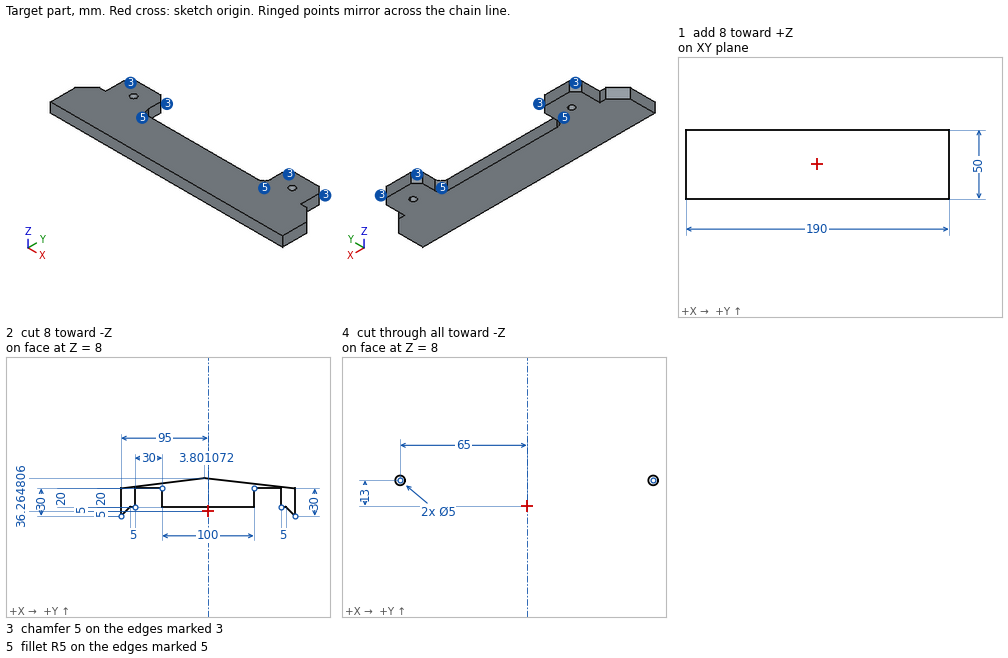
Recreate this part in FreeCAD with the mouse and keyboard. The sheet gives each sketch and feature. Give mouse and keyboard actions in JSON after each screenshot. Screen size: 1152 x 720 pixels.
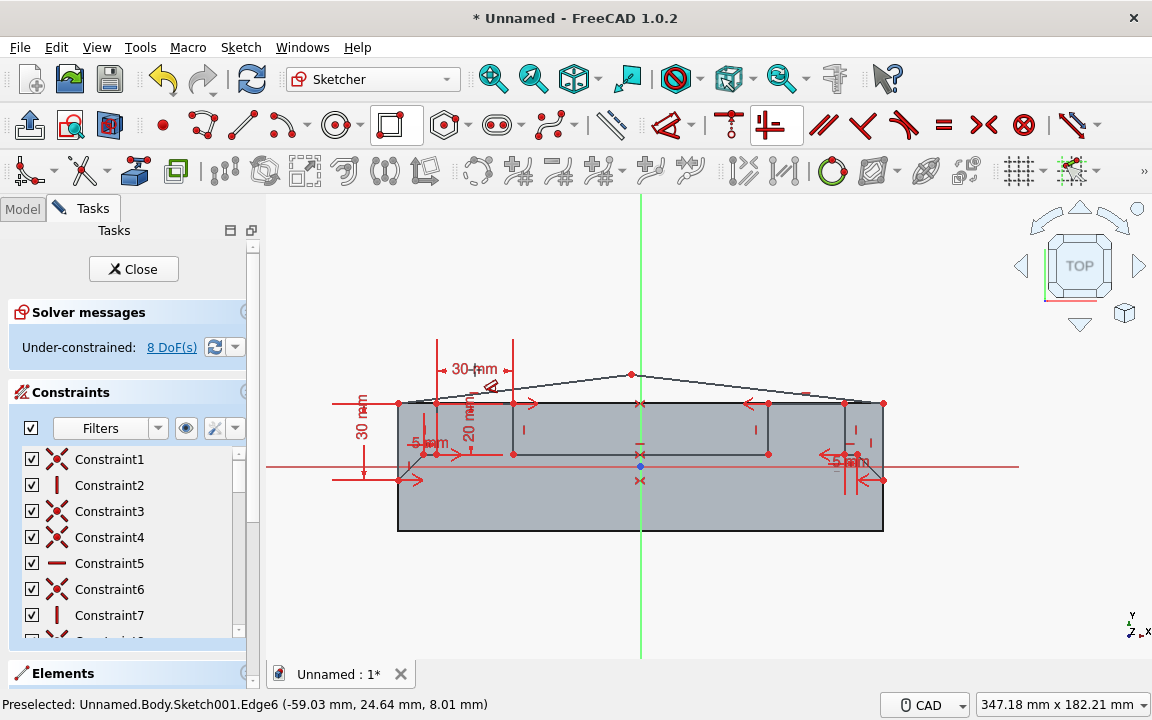
{"action": "left_click", "coordinate": [513, 419]}
{"action": "left_click", "coordinate": [547, 429]}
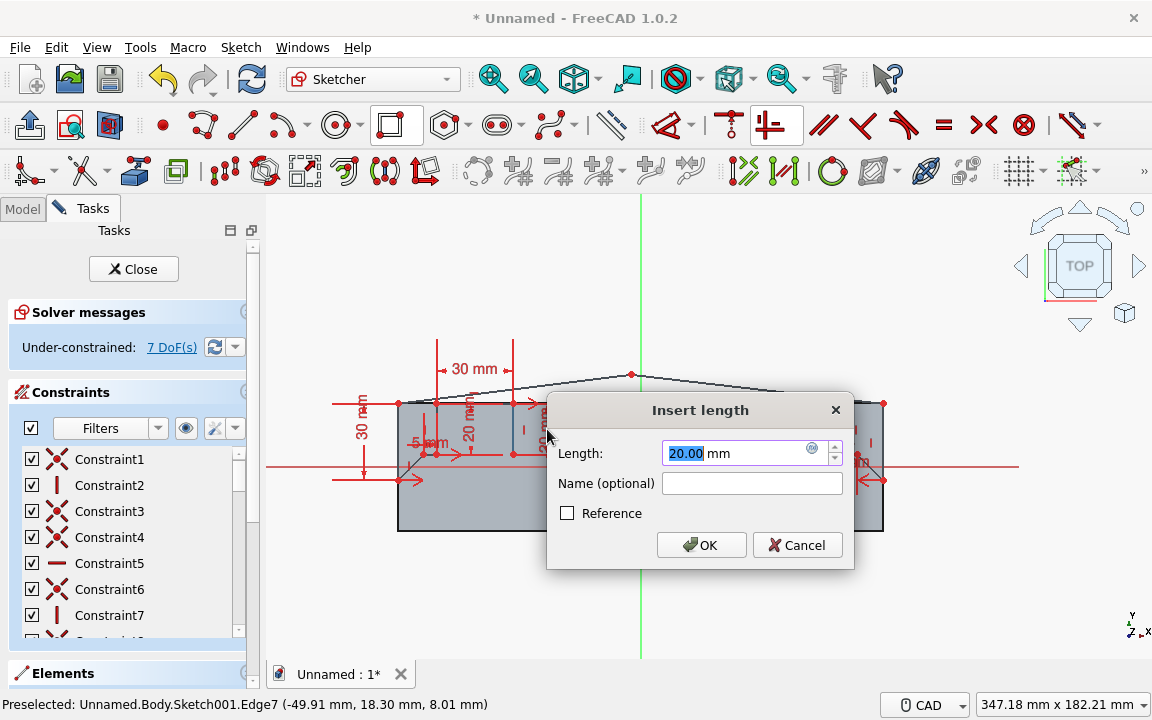
{"action": "type", "text": "20"}
{"action": "key", "text": "Return"}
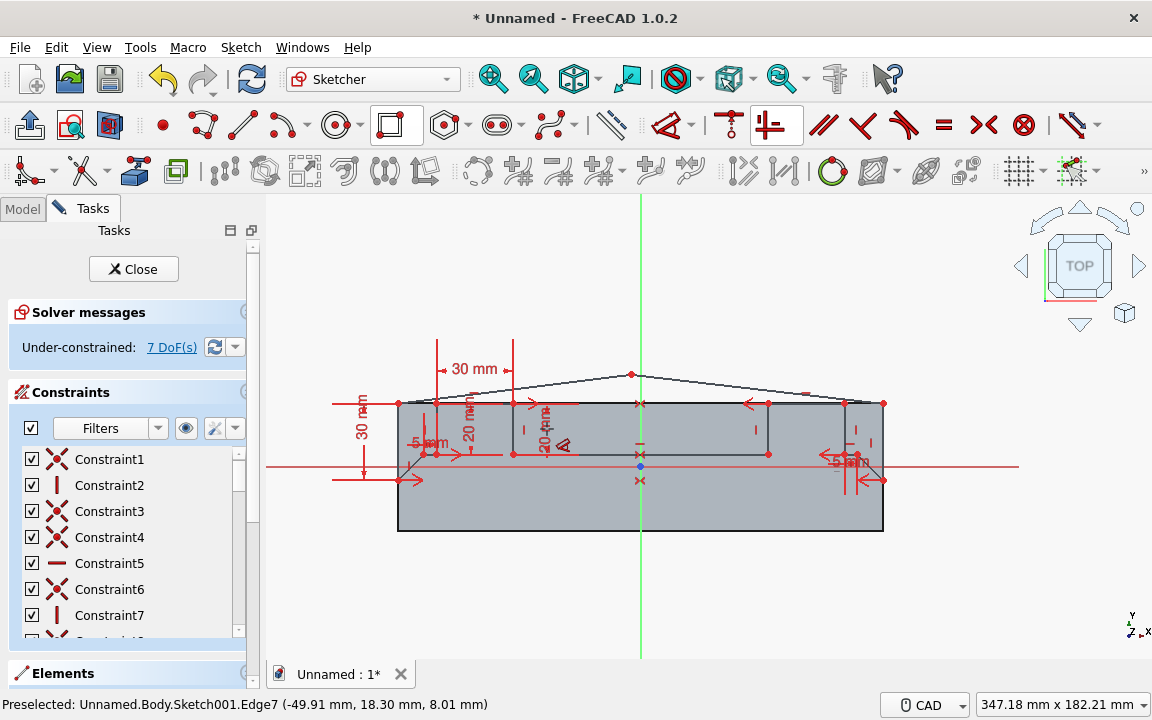
{"action": "scroll", "coordinate": [883, 457], "scroll_direction": "up", "scroll_amount": 2}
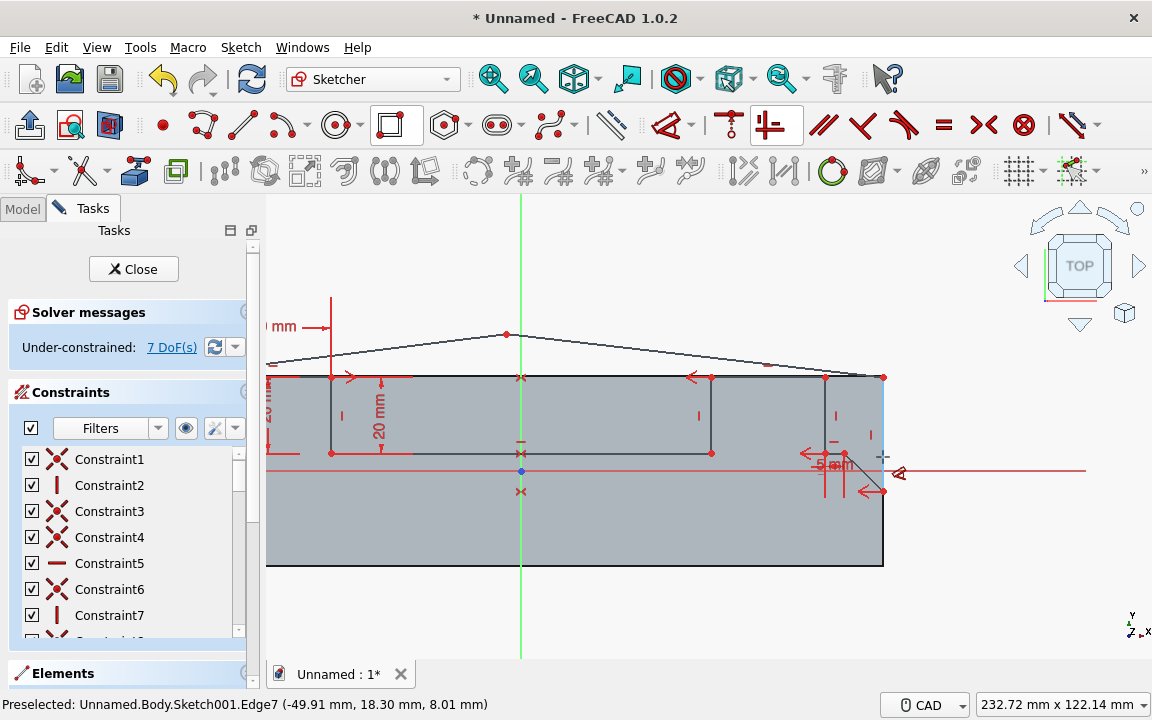
{"action": "left_click", "coordinate": [883, 457]}
{"action": "left_click", "coordinate": [917, 435]}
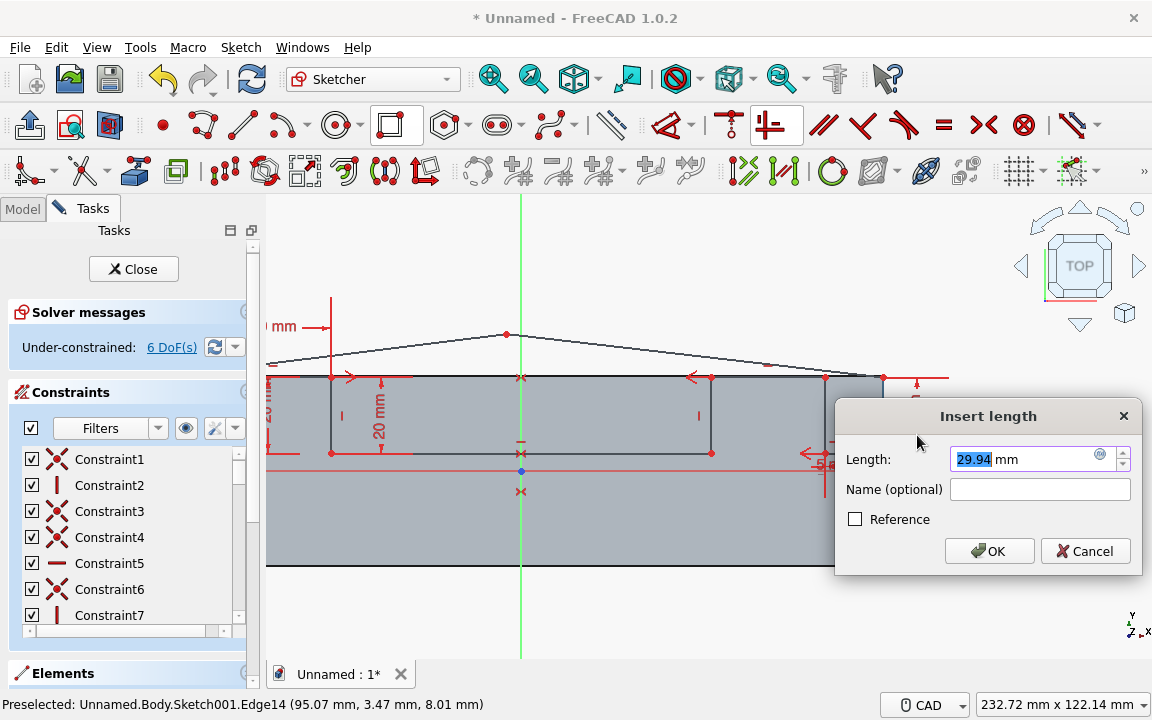
{"action": "type", "text": "30"}
{"action": "key", "text": "Return"}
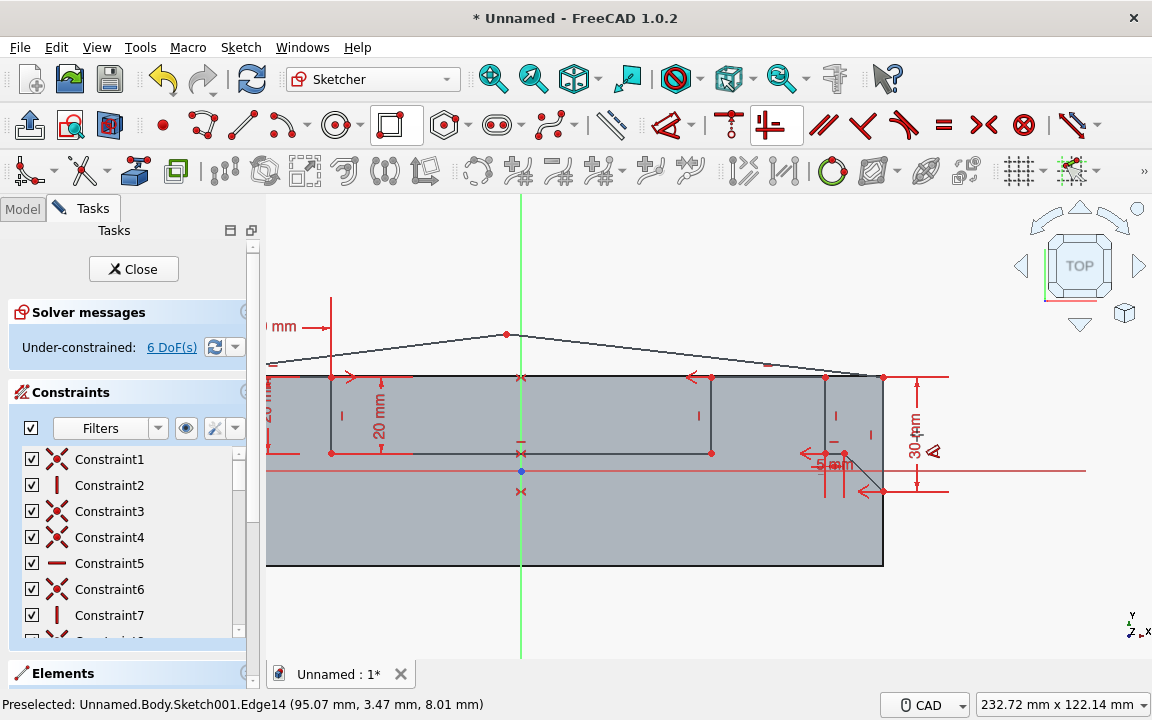
{"action": "scroll", "coordinate": [883, 457], "scroll_direction": "down", "scroll_amount": 2}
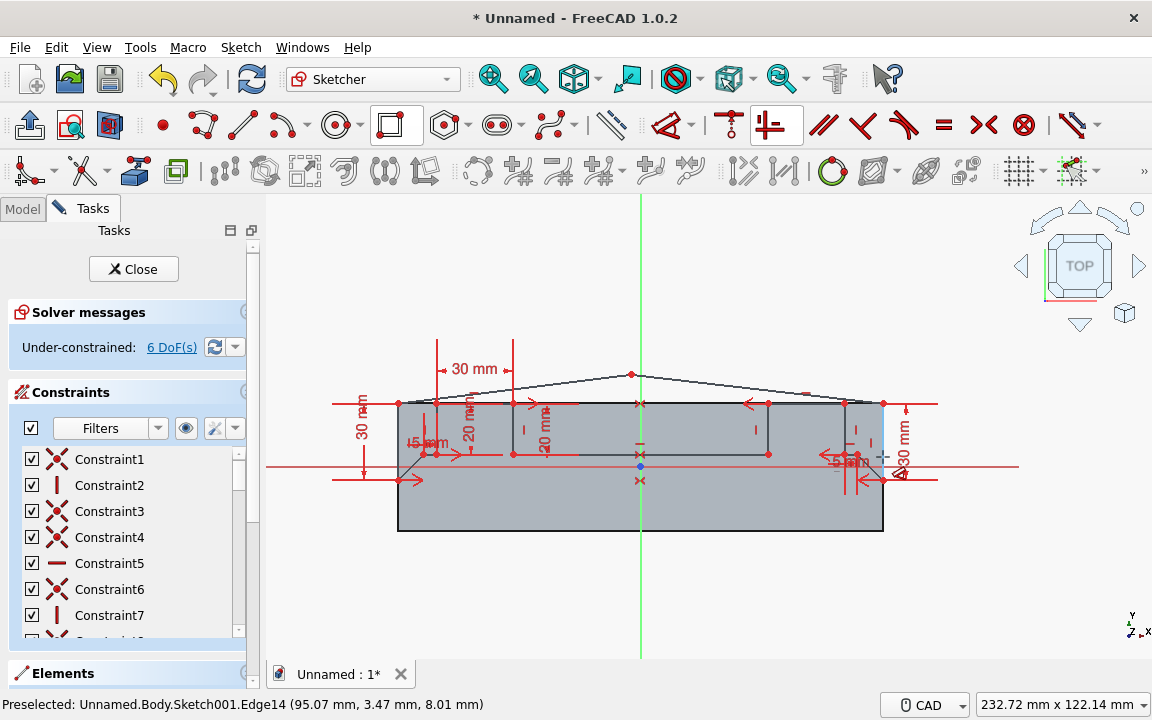
{"action": "scroll", "coordinate": [398, 480], "scroll_direction": "up", "scroll_amount": 6}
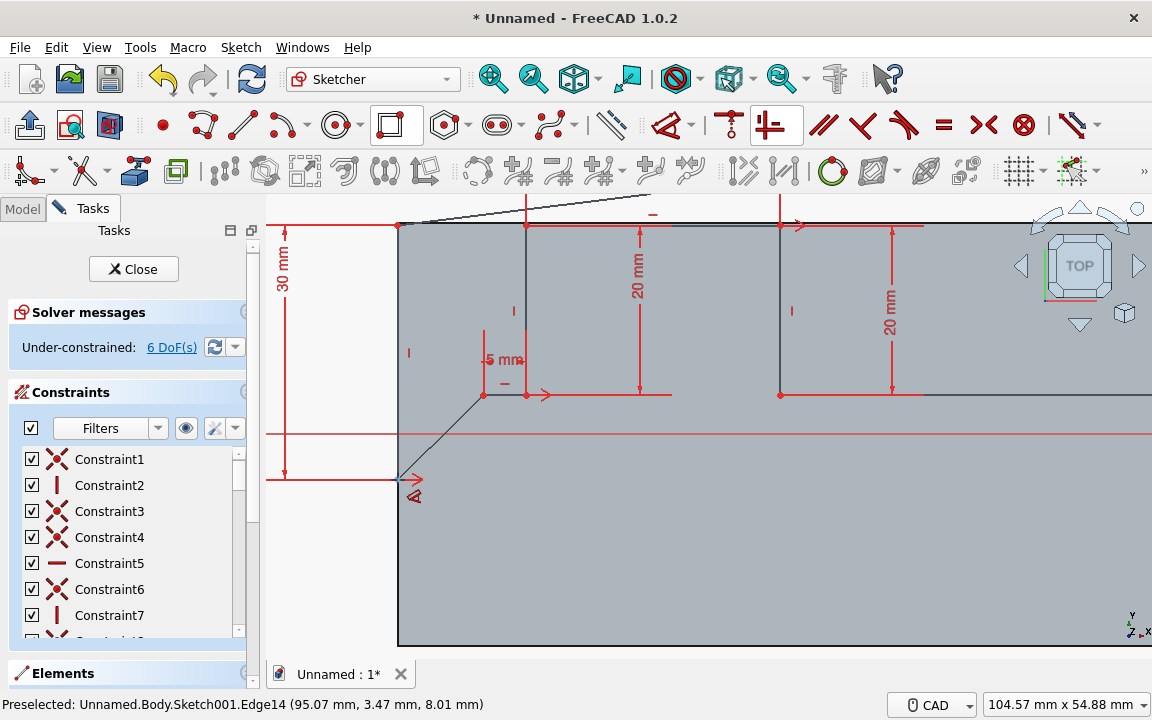
{"action": "left_click", "coordinate": [398, 480]}
{"action": "left_click", "coordinate": [364, 457]}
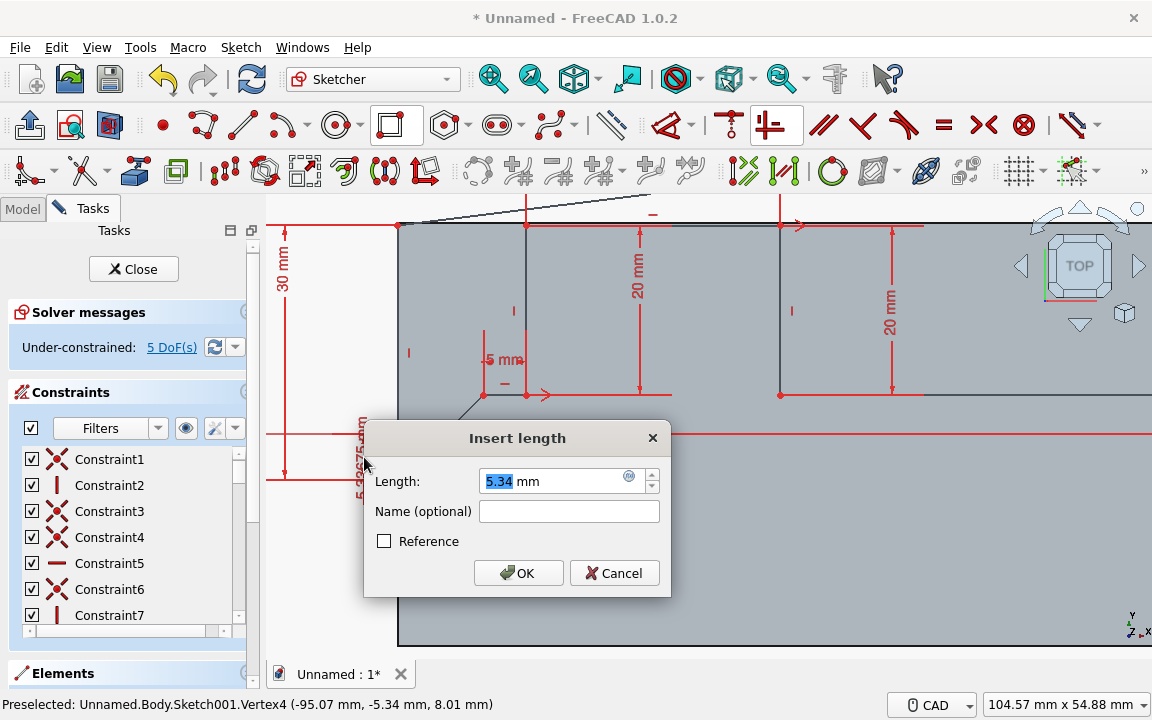
{"action": "type", "text": "5"}
{"action": "key", "text": "Return"}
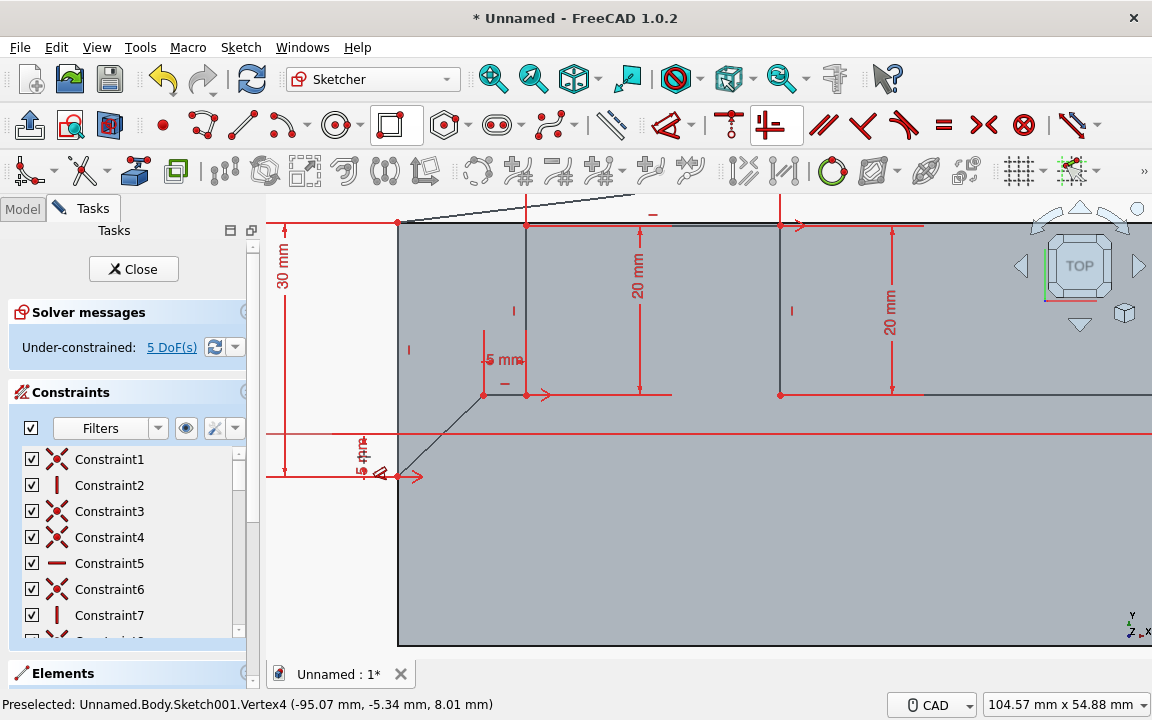
{"action": "left_click", "coordinate": [484, 395]}
{"action": "left_click", "coordinate": [450, 406]}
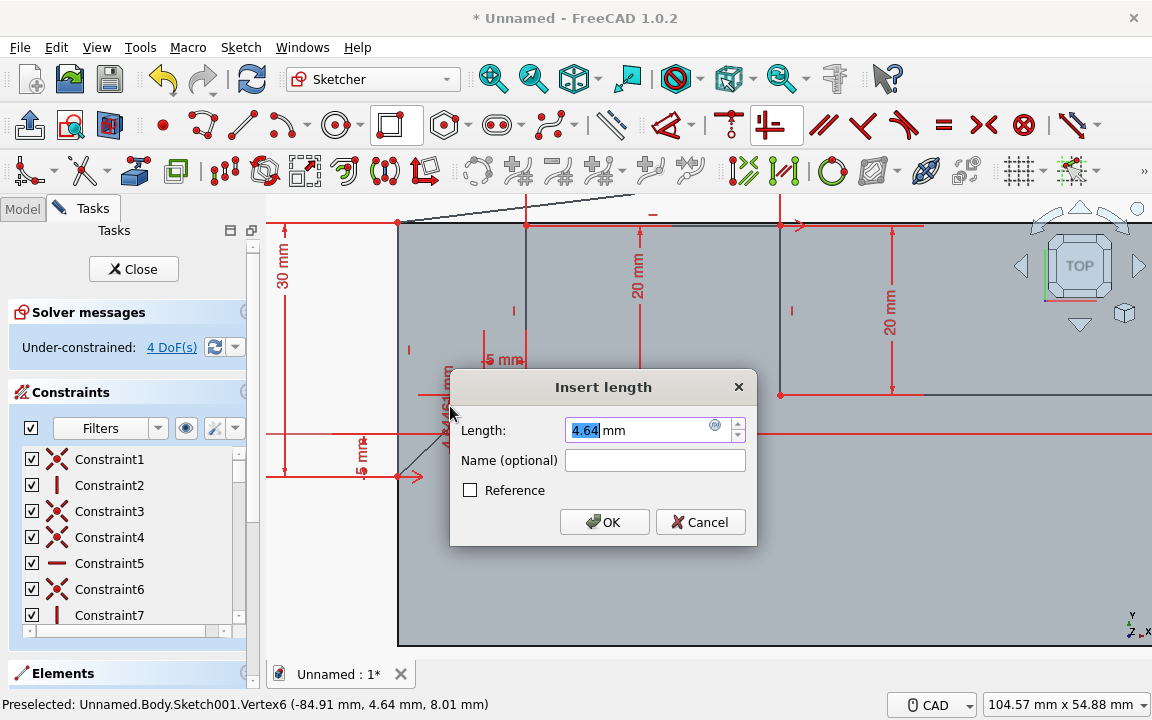
{"action": "type", "text": "5"}
{"action": "key", "text": "Return"}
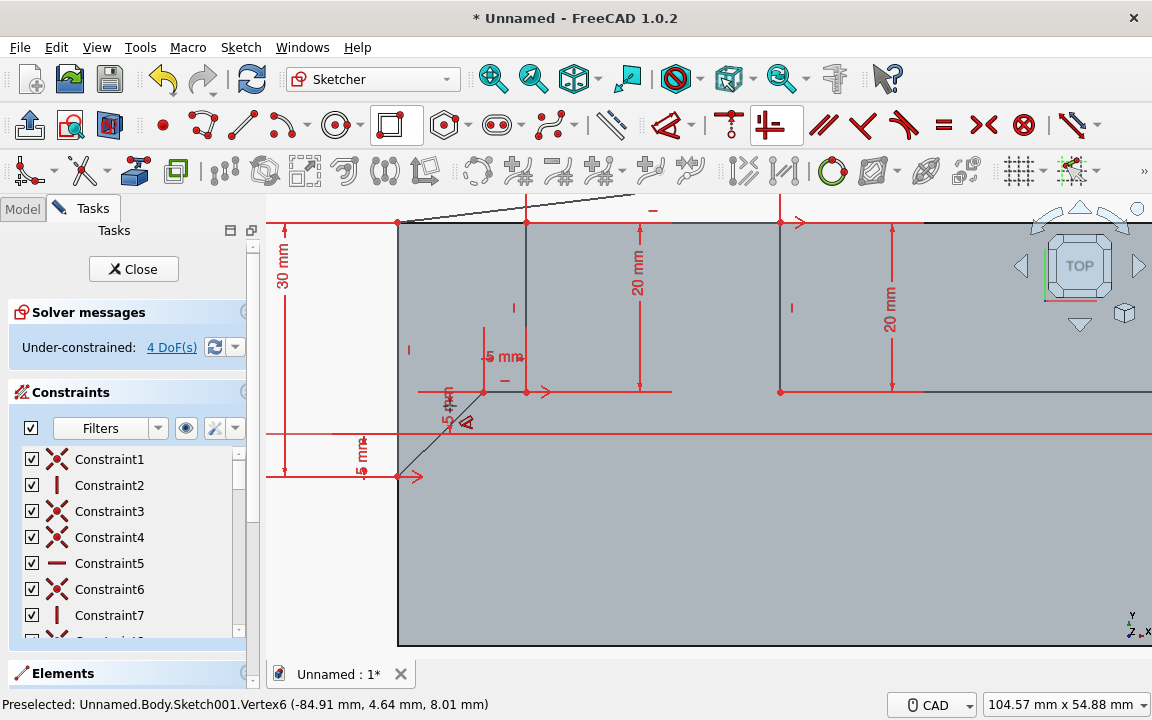
{"action": "left_click", "coordinate": [950, 392]}
{"action": "left_click", "coordinate": [884, 358]}